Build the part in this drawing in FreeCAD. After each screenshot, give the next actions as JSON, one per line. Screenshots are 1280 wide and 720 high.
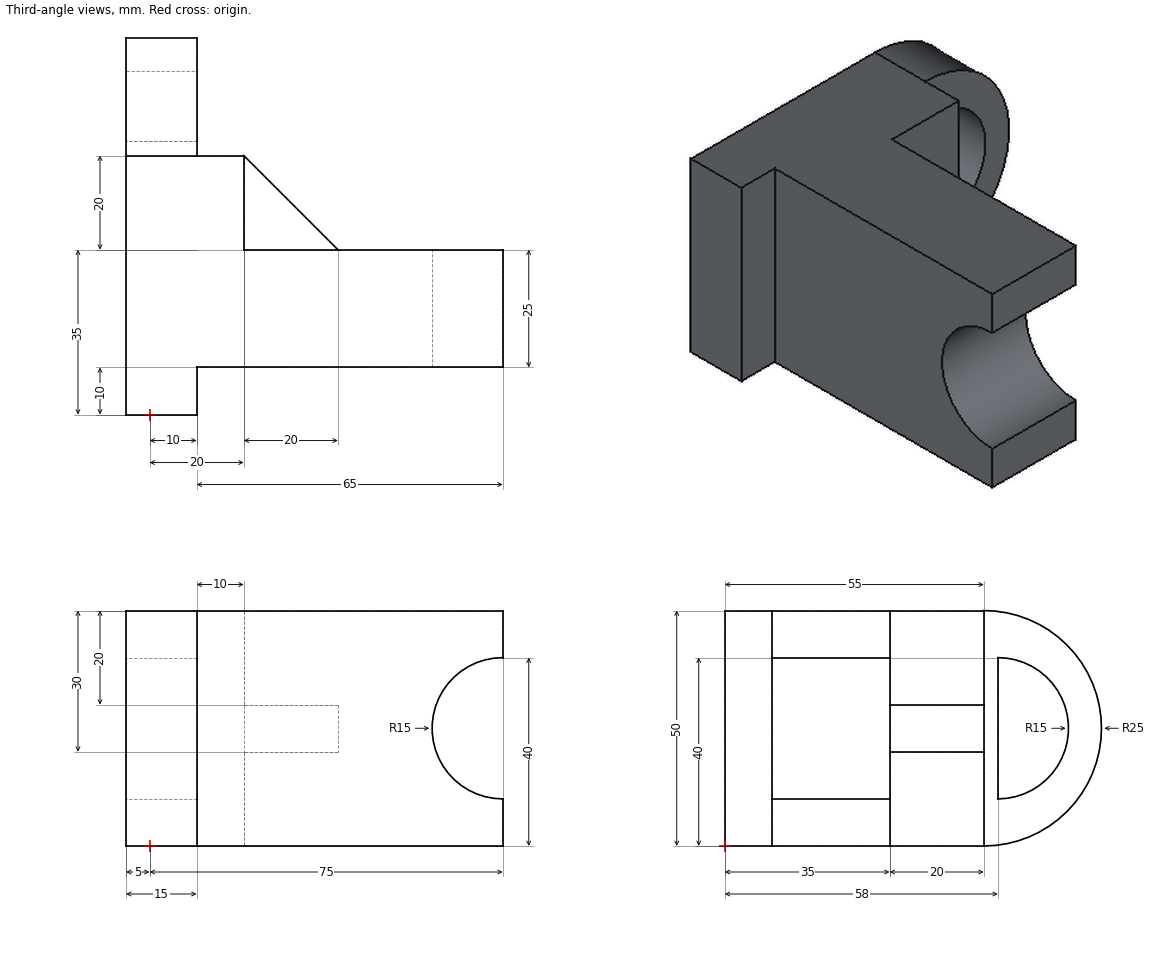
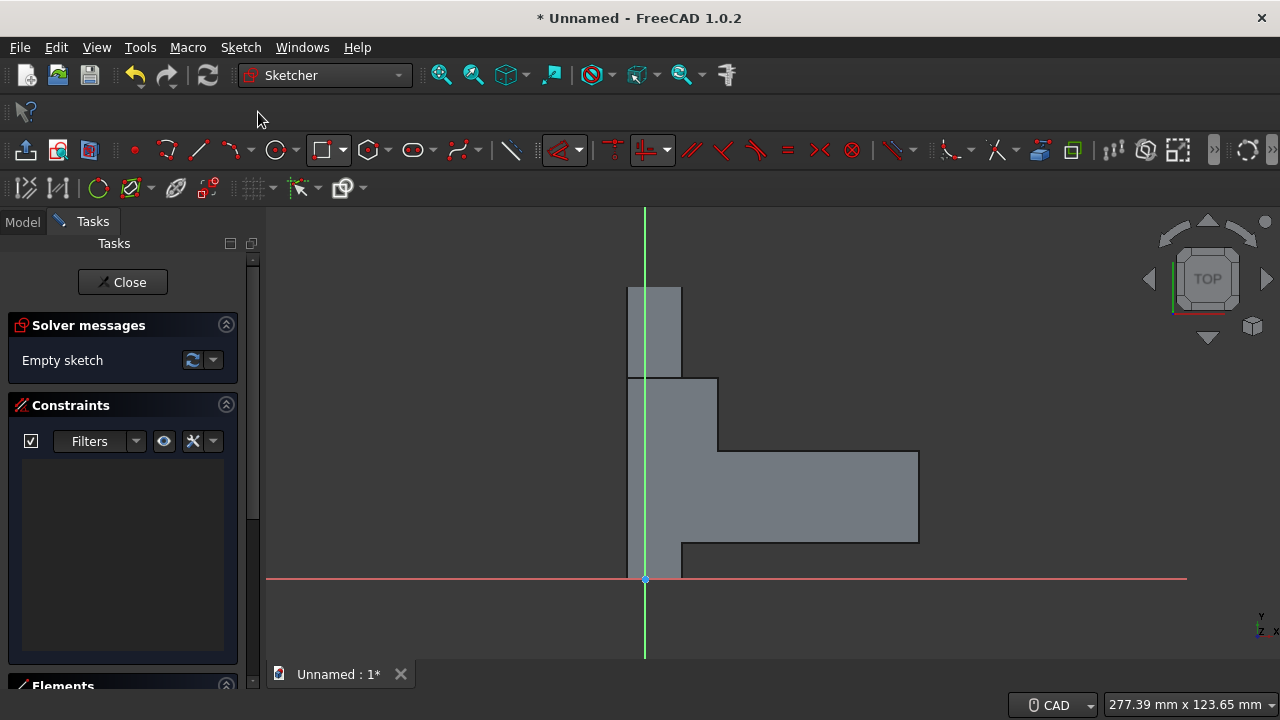
{"action": "scroll", "coordinate": [771, 409], "scroll_direction": "up", "scroll_amount": 7}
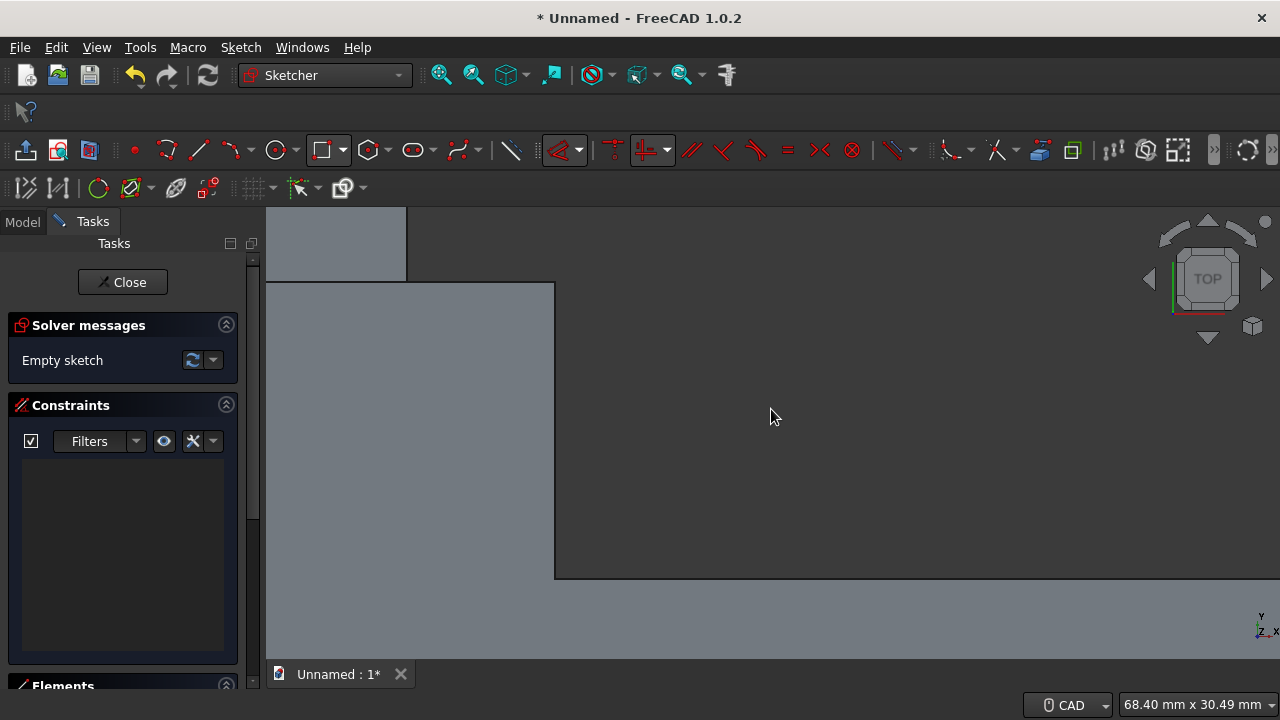
{"action": "left_click", "coordinate": [168, 150]}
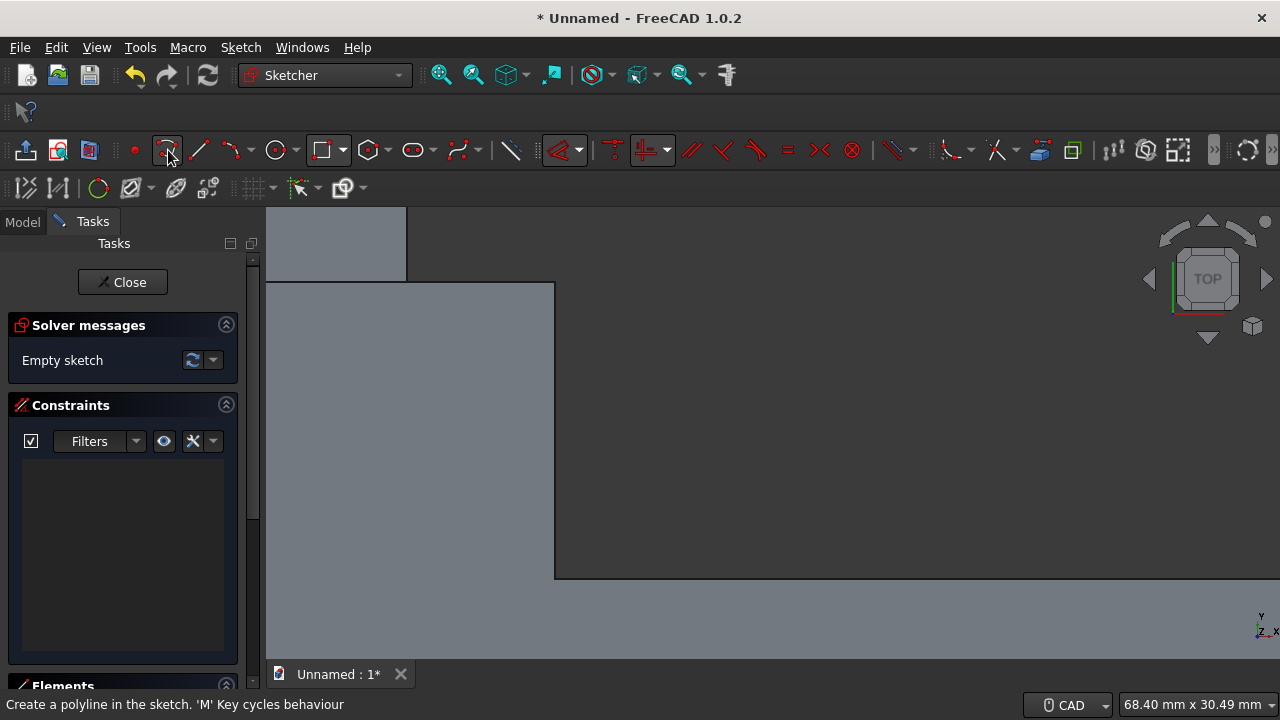
{"action": "left_click", "coordinate": [555, 579]}
{"action": "left_click", "coordinate": [852, 579]}
{"action": "left_click", "coordinate": [555, 282]}
{"action": "left_click", "coordinate": [555, 580]}
{"action": "key", "text": "Escape"}
{"action": "key", "text": "Escape"}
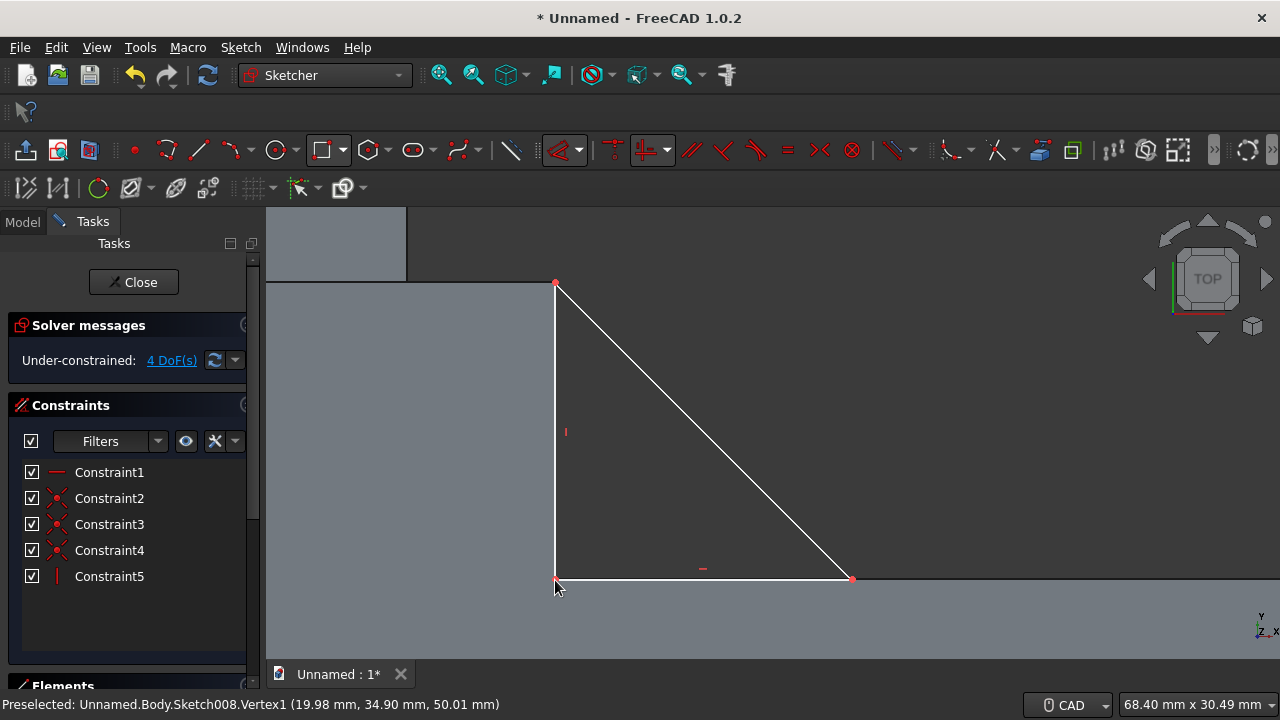
{"action": "left_click", "coordinate": [644, 580]}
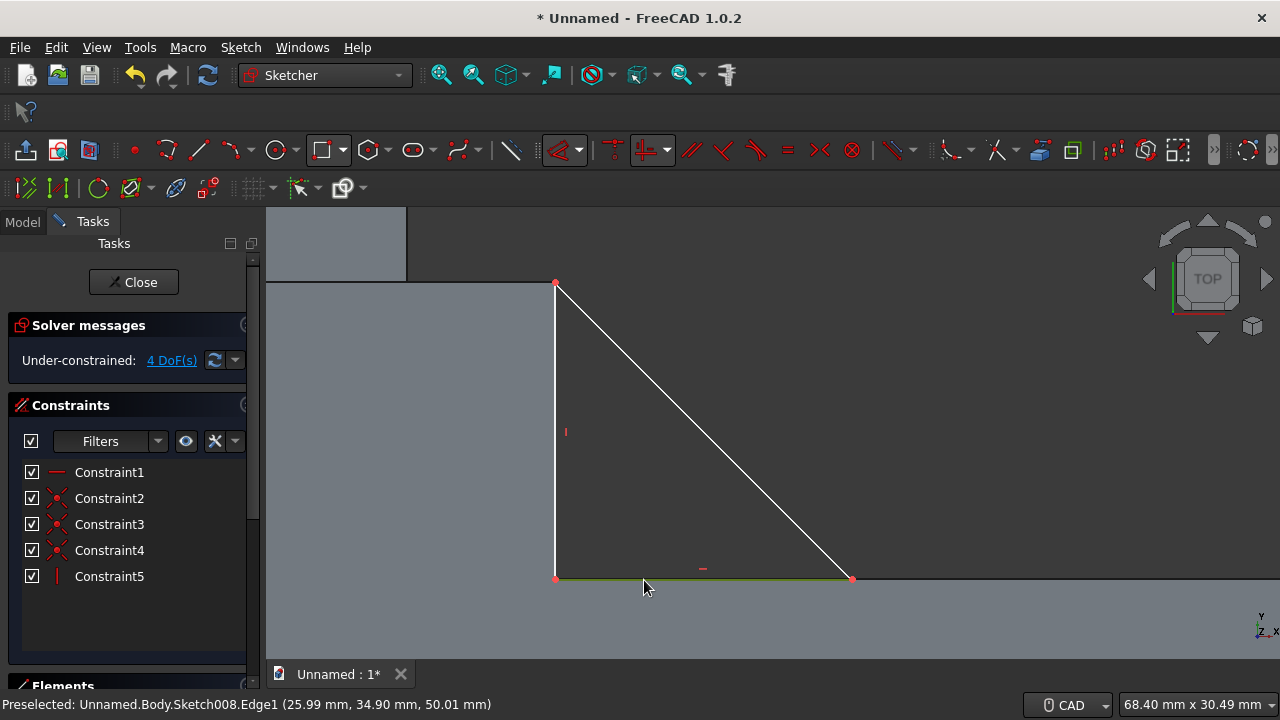
{"action": "key", "text": "l"}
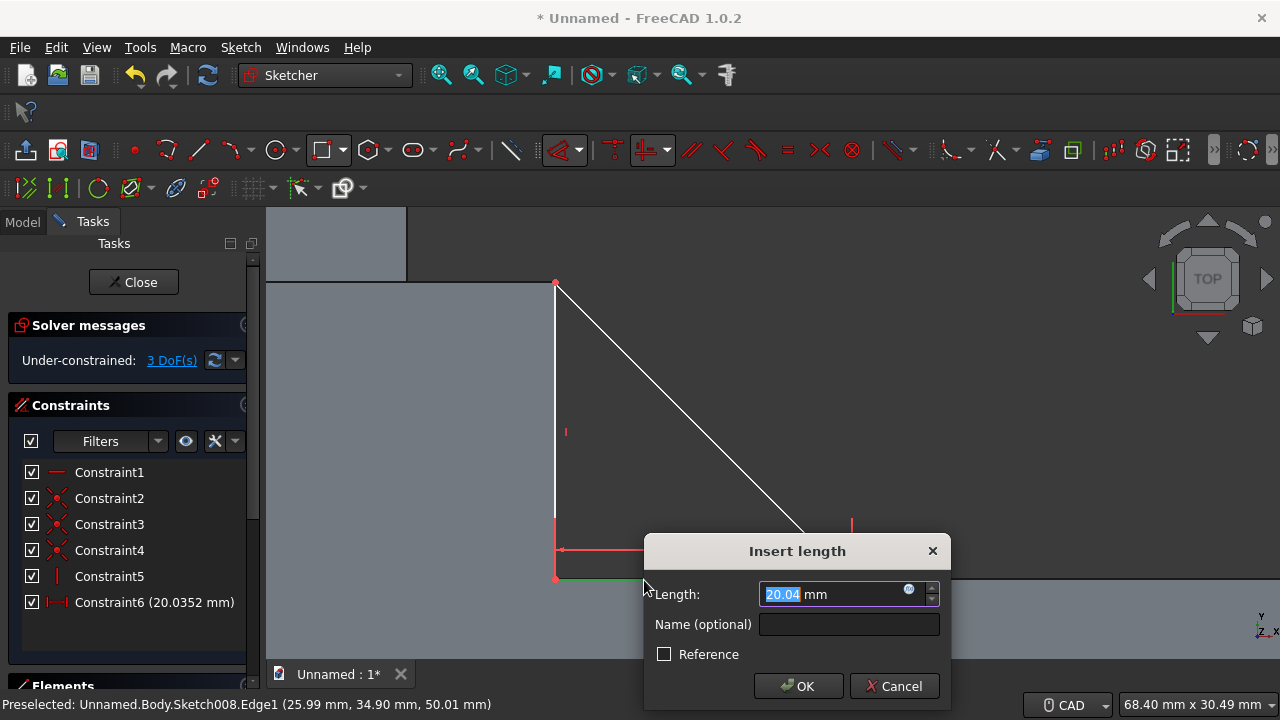
{"action": "type", "text": "20"}
{"action": "key", "text": "Return"}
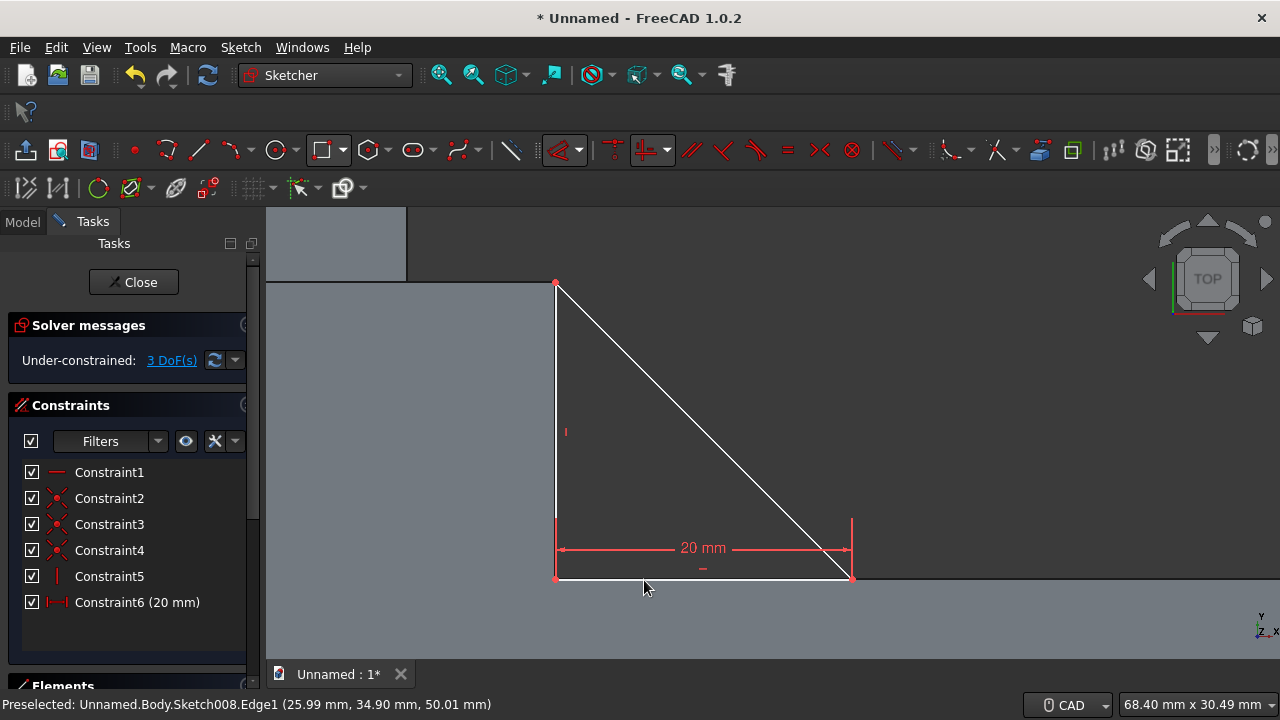
{"action": "left_click", "coordinate": [556, 372]}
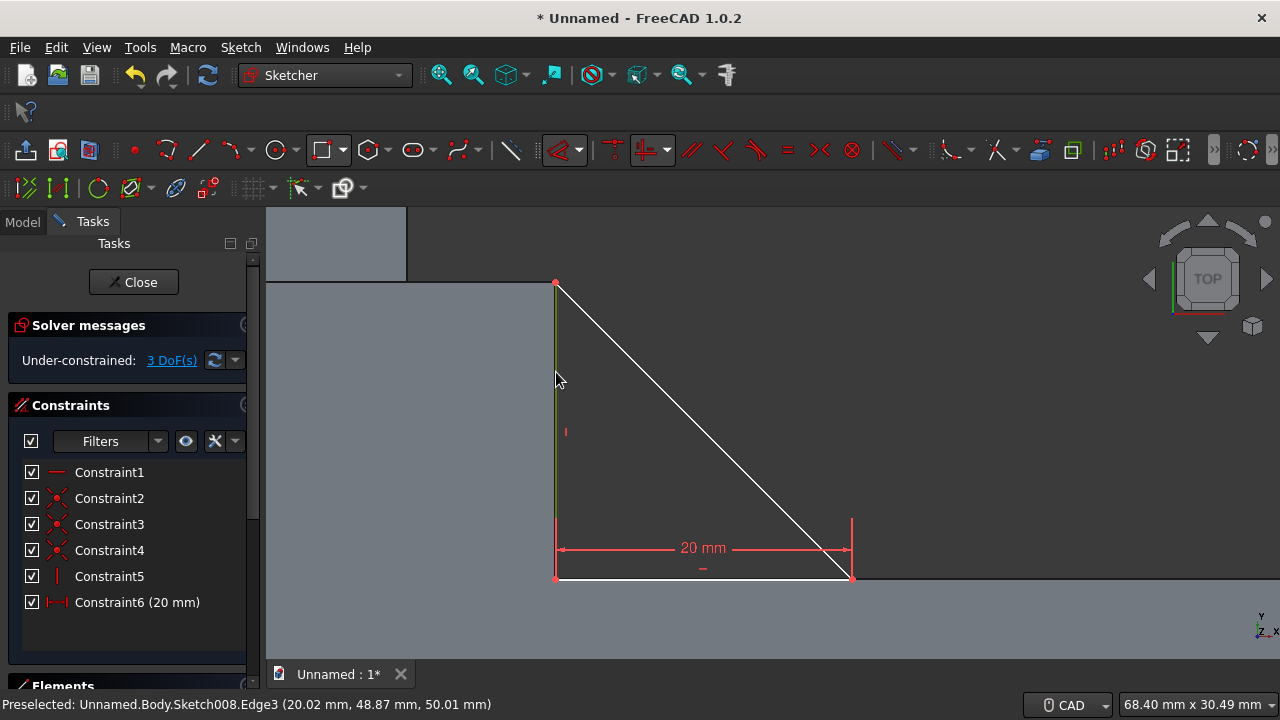
{"action": "key", "text": "i"}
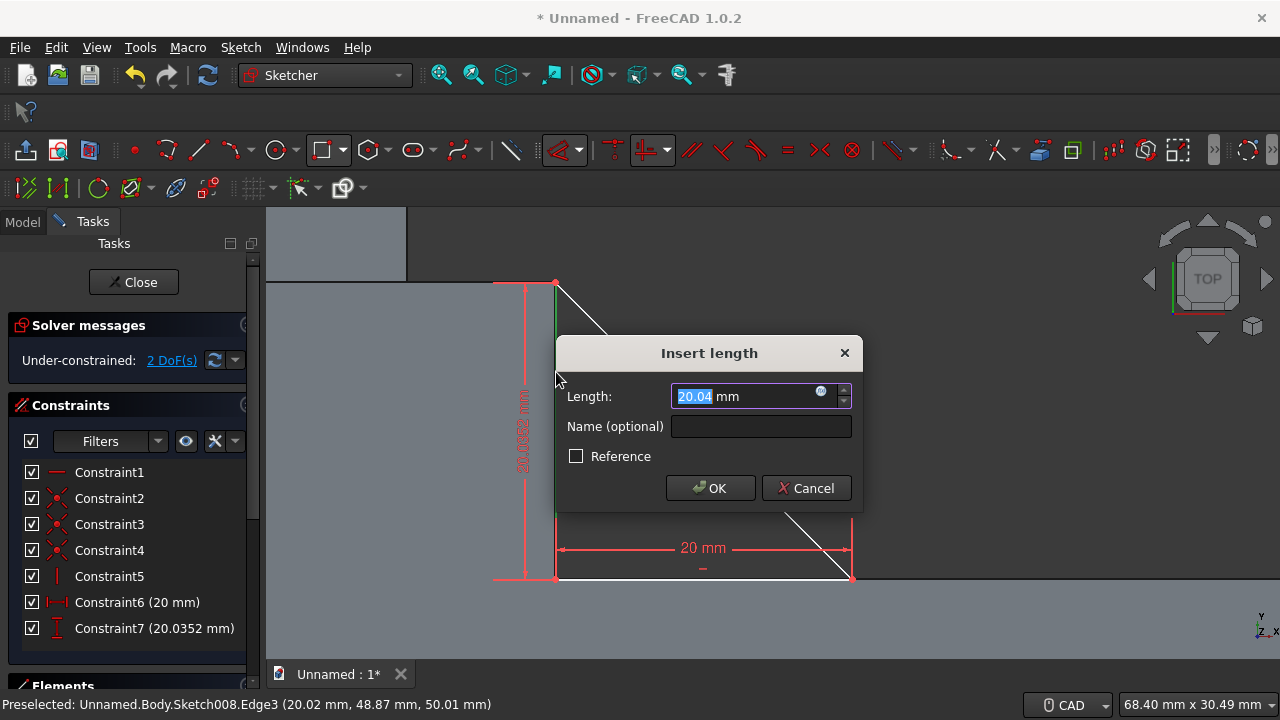
{"action": "type", "text": "20"}
{"action": "key", "text": "Return"}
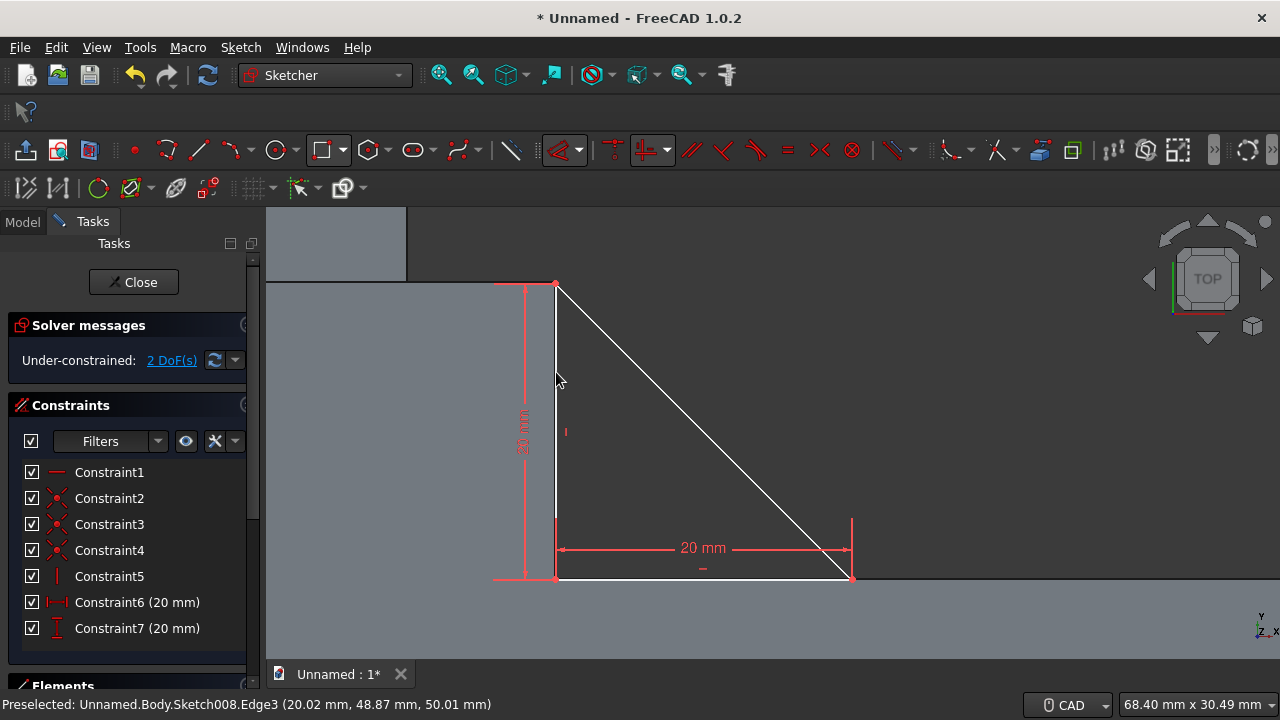
{"action": "left_click", "coordinate": [556, 580]}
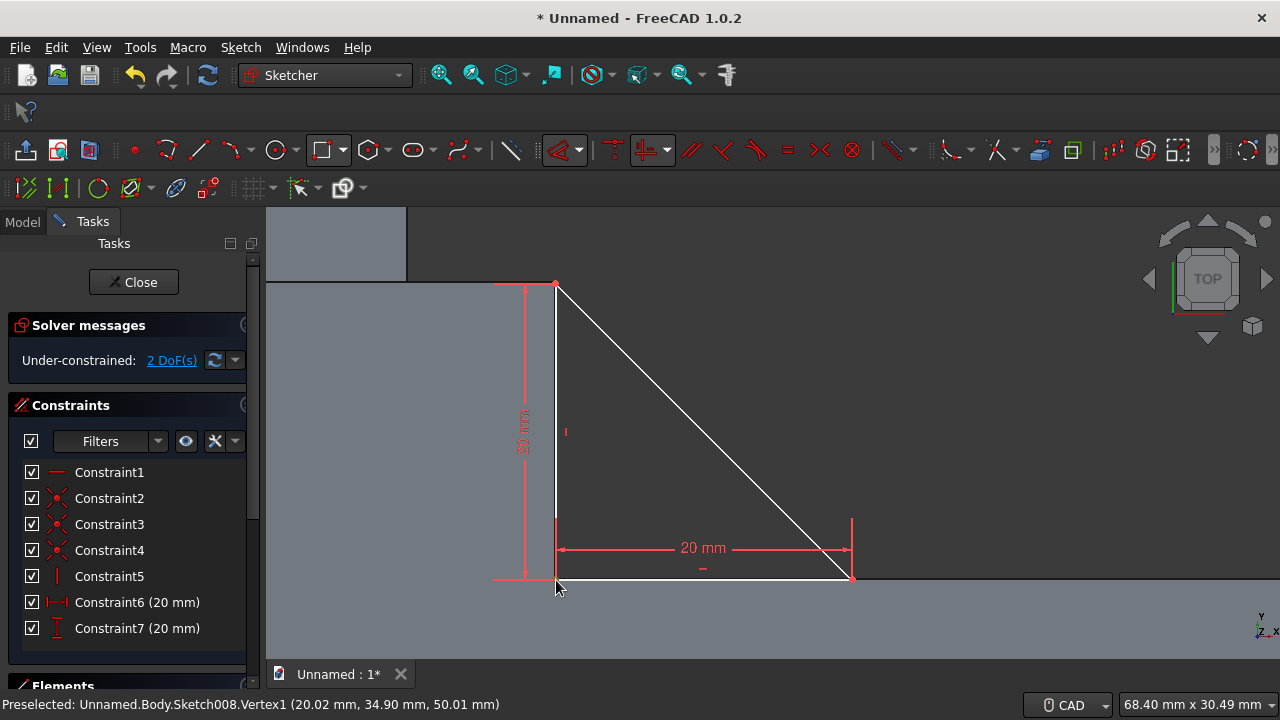
{"action": "key", "text": "l"}